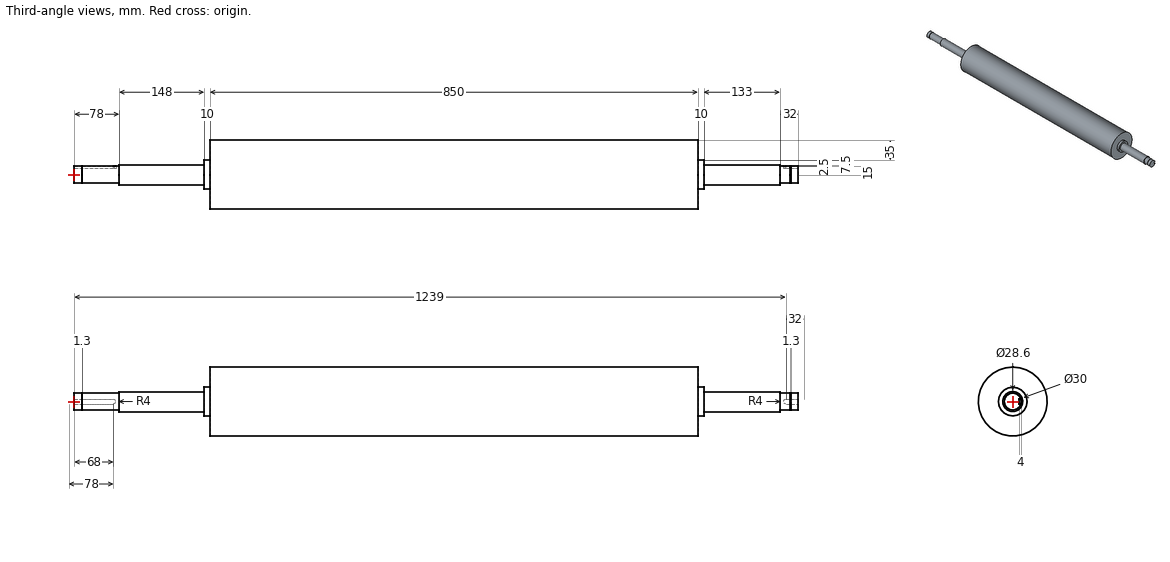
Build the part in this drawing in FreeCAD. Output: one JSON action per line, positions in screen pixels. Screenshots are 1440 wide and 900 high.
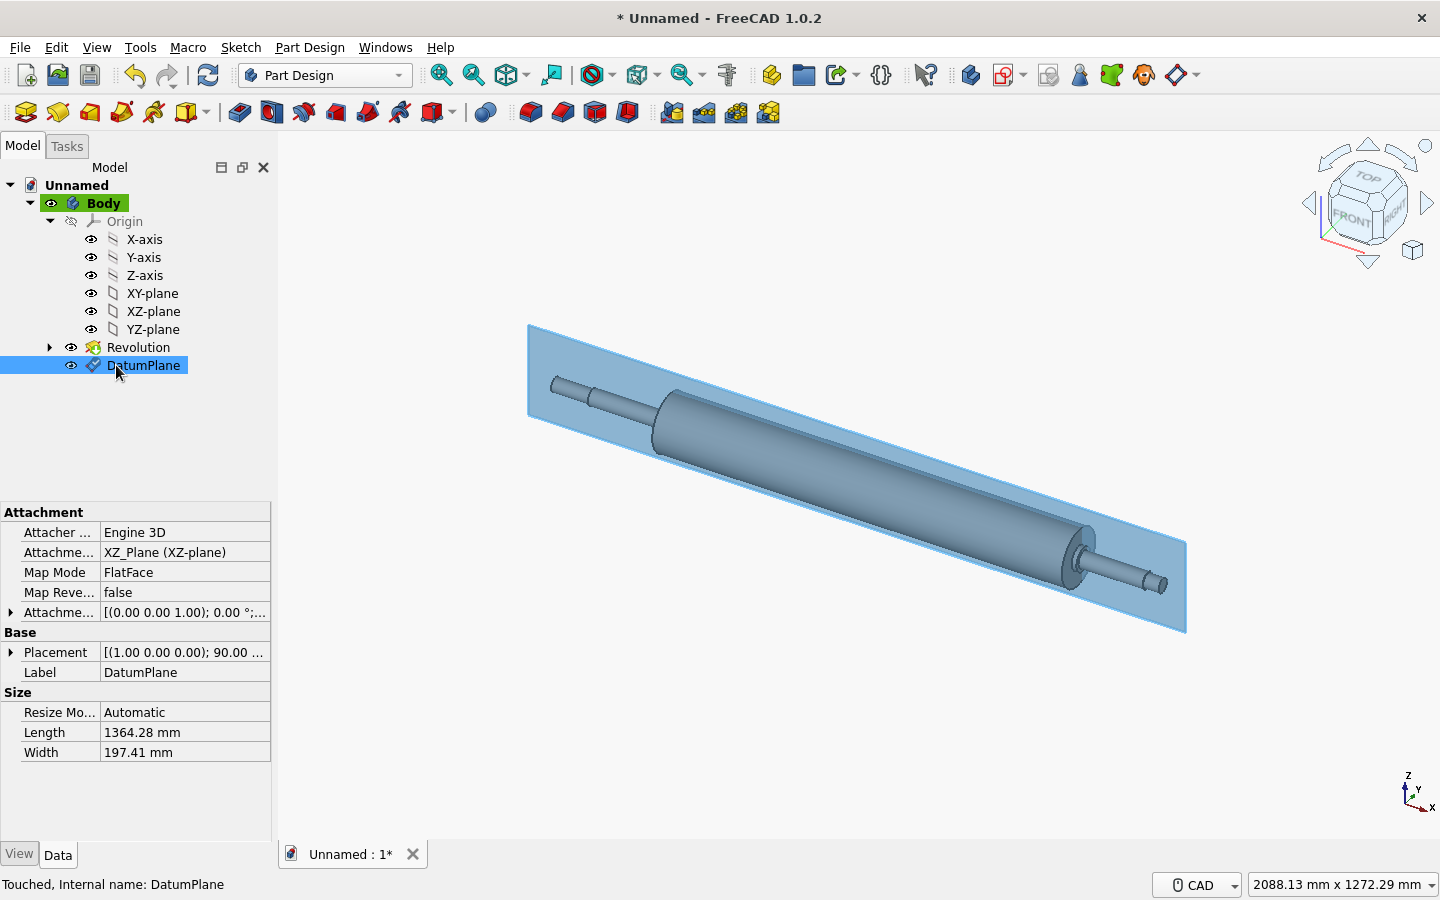
{"action": "left_click", "coordinate": [1004, 76]}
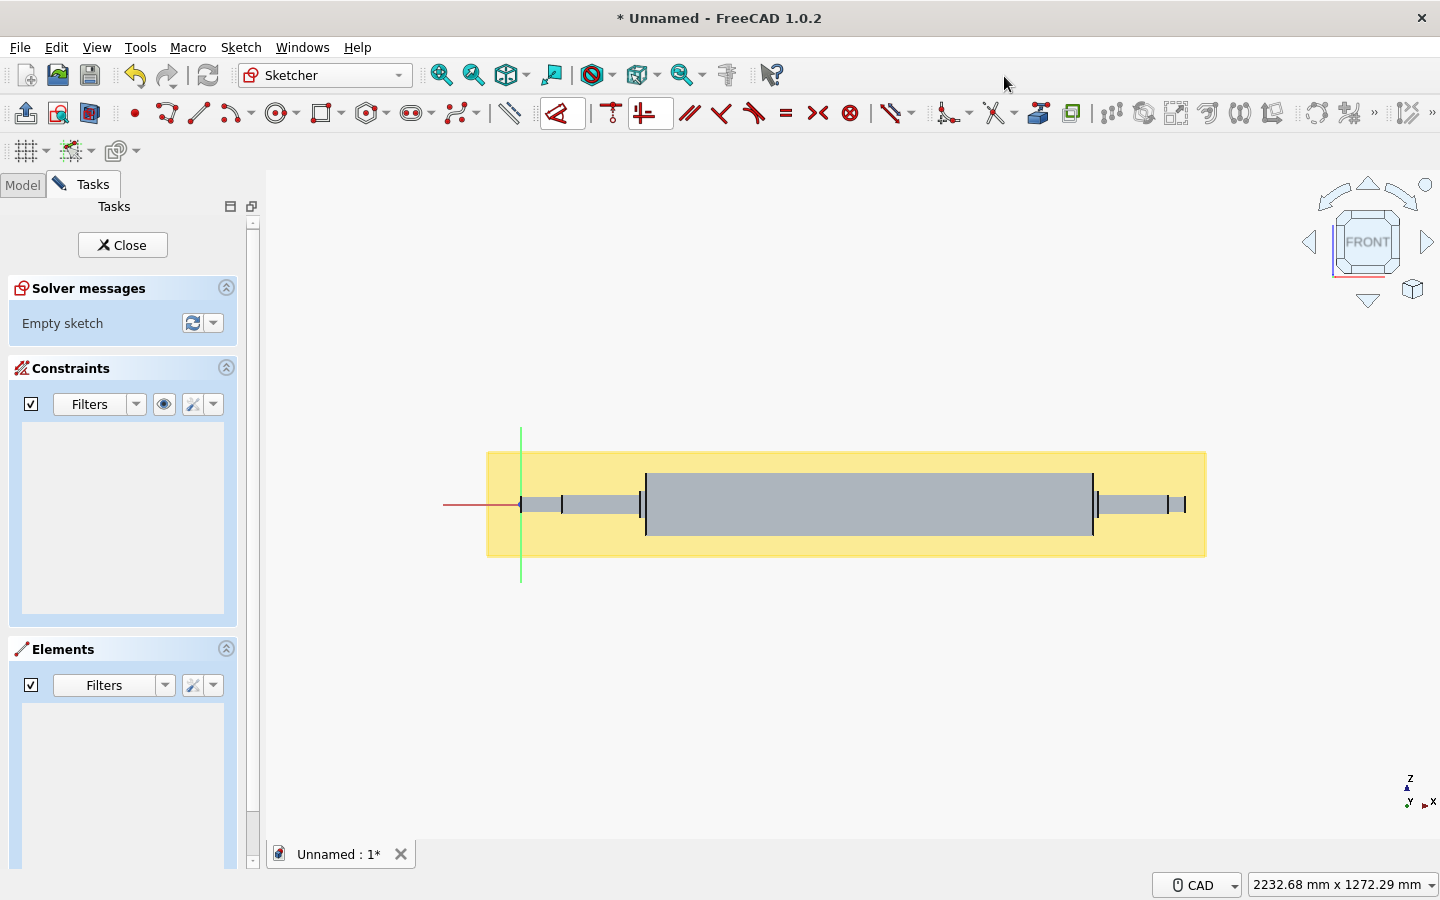
{"action": "left_click", "coordinate": [90, 114]}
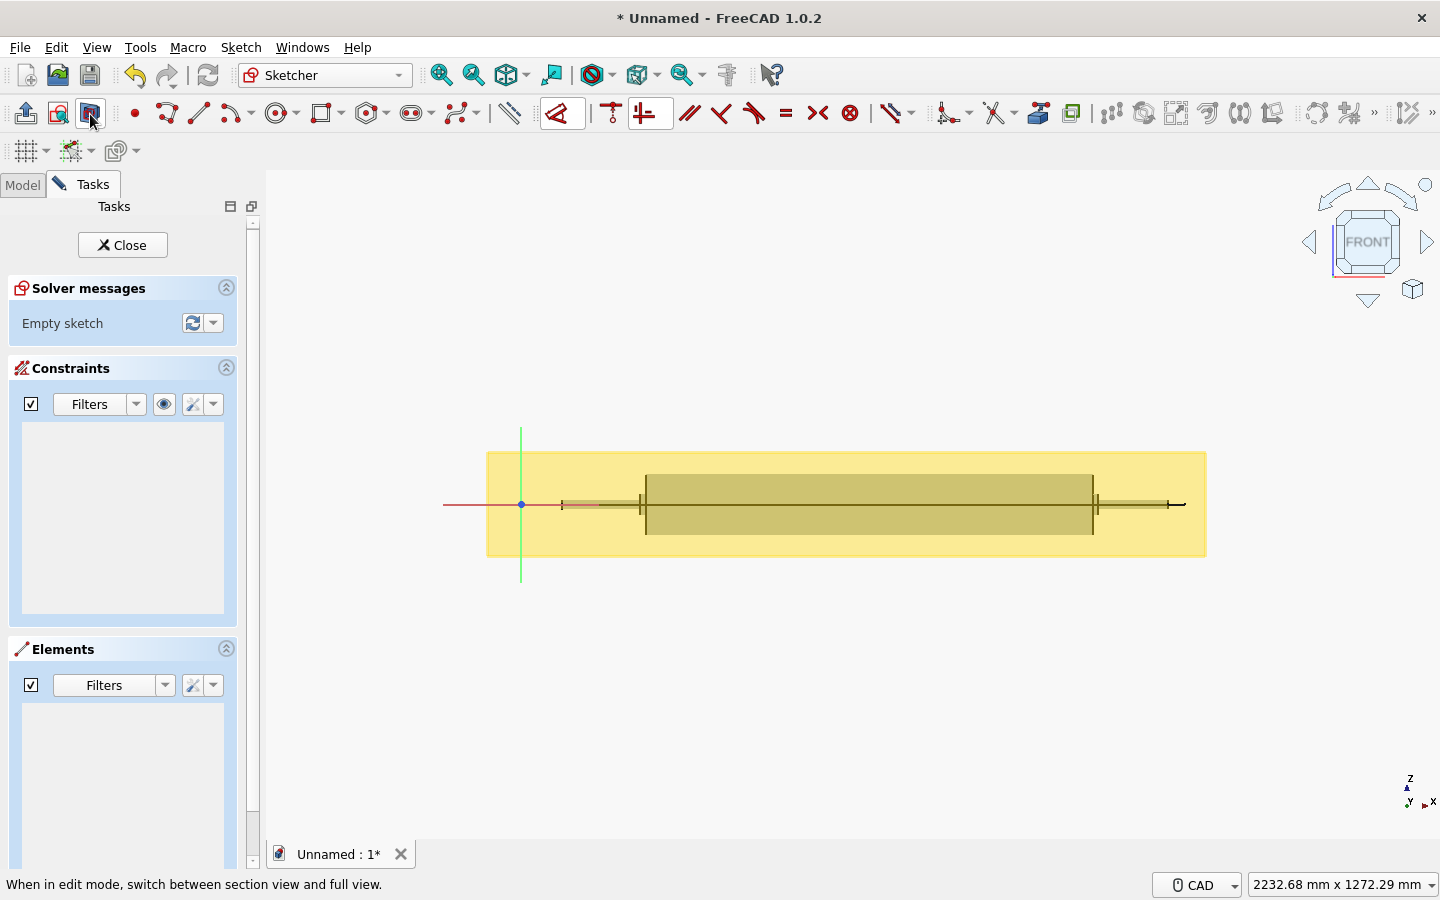
{"action": "scroll", "coordinate": [522, 505], "scroll_direction": "up", "scroll_amount": 14}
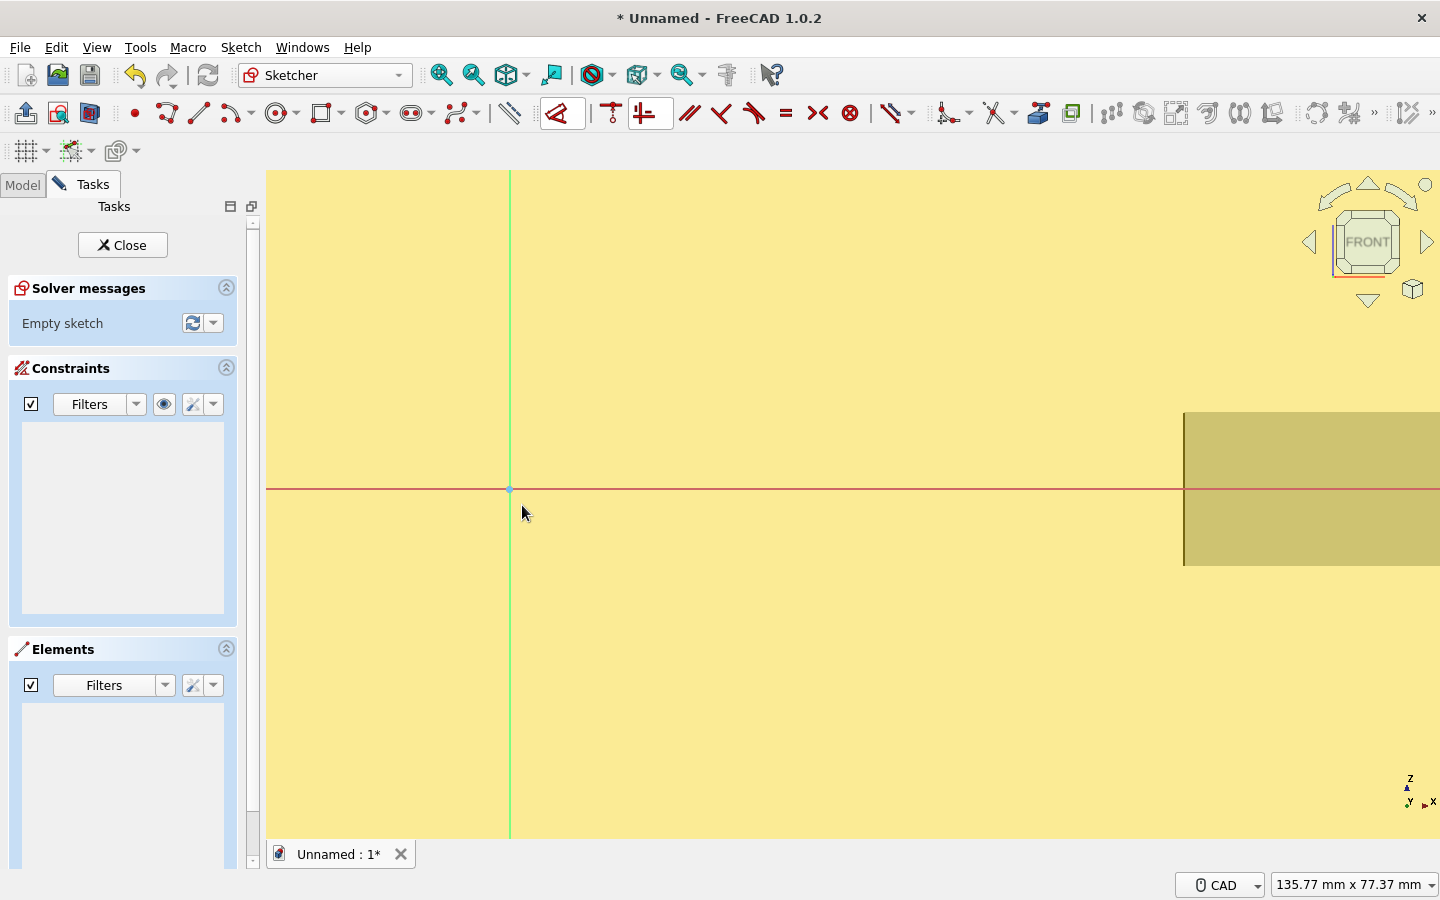
{"action": "key", "text": "g m"}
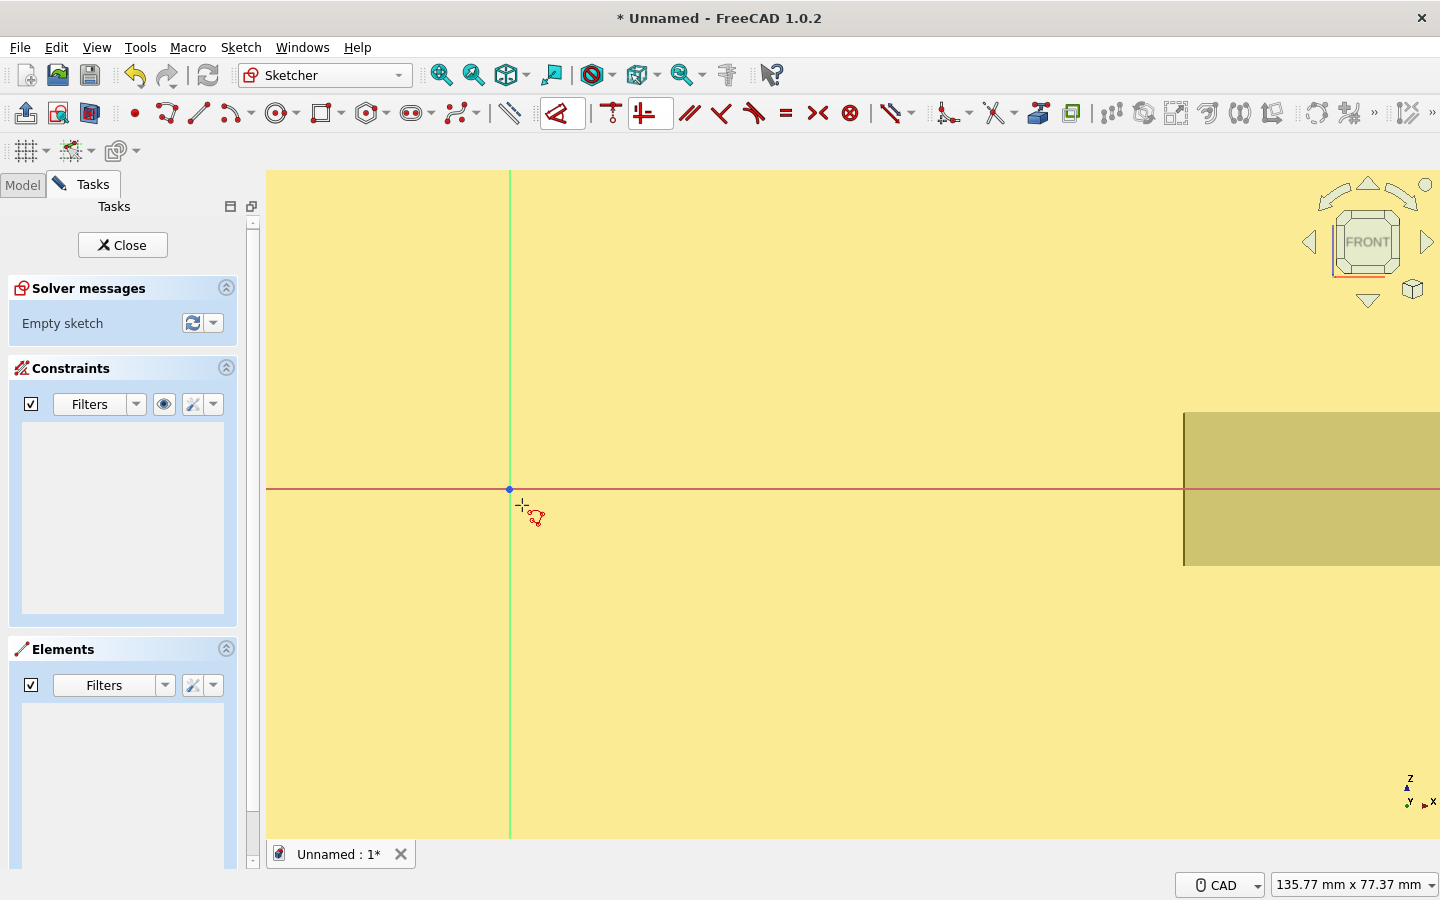
{"action": "left_click", "coordinate": [1098, 524]}
{"action": "left_click", "coordinate": [423, 524]}
{"action": "left_click", "coordinate": [423, 454]}
{"action": "left_click", "coordinate": [1098, 454]}
{"action": "right_click", "coordinate": [1098, 454]}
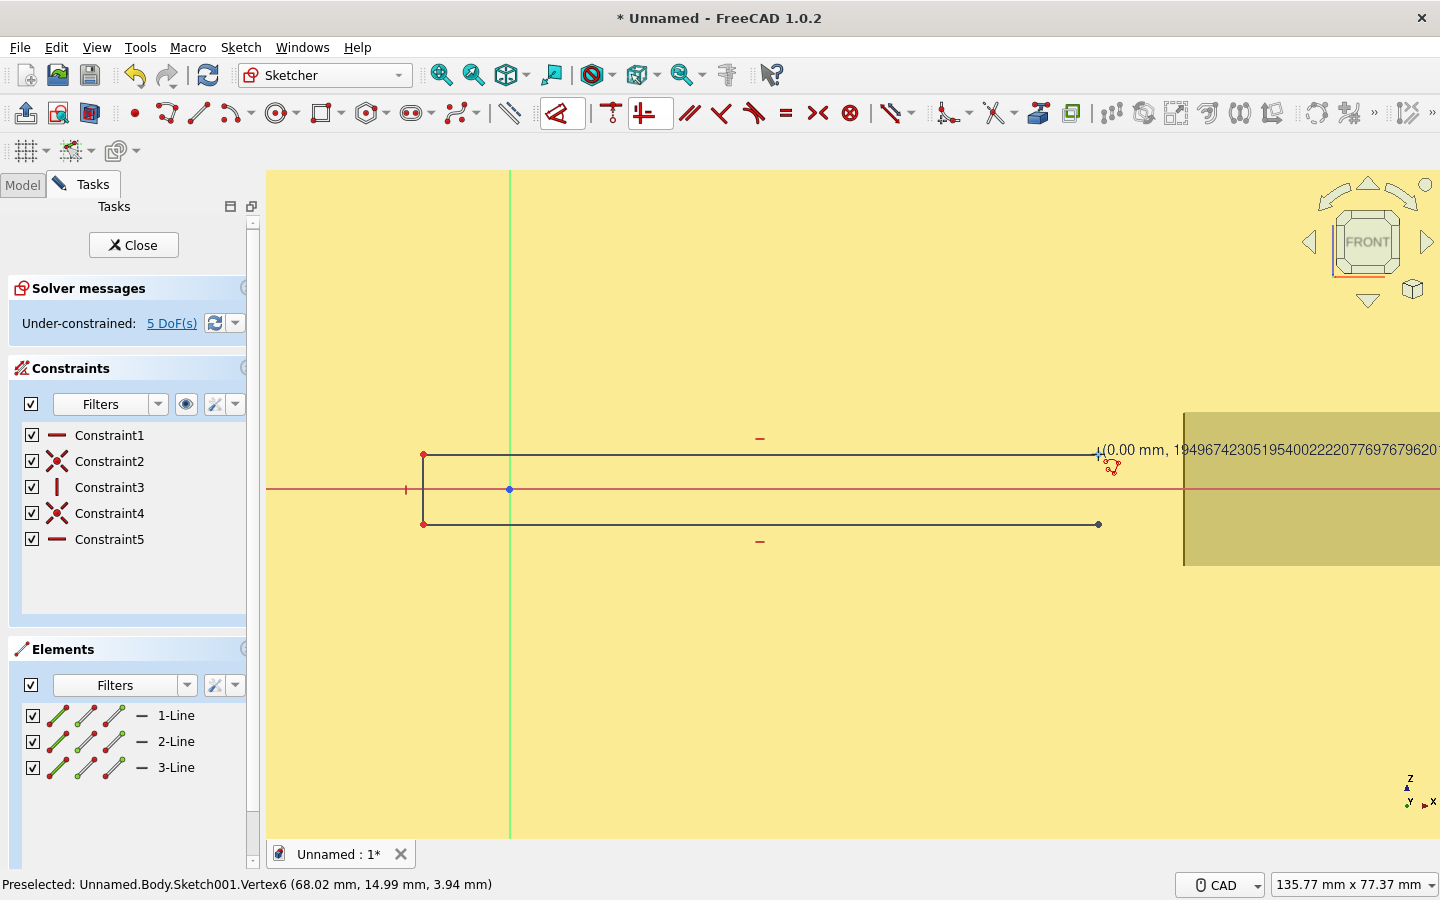
{"action": "left_click", "coordinate": [254, 114]}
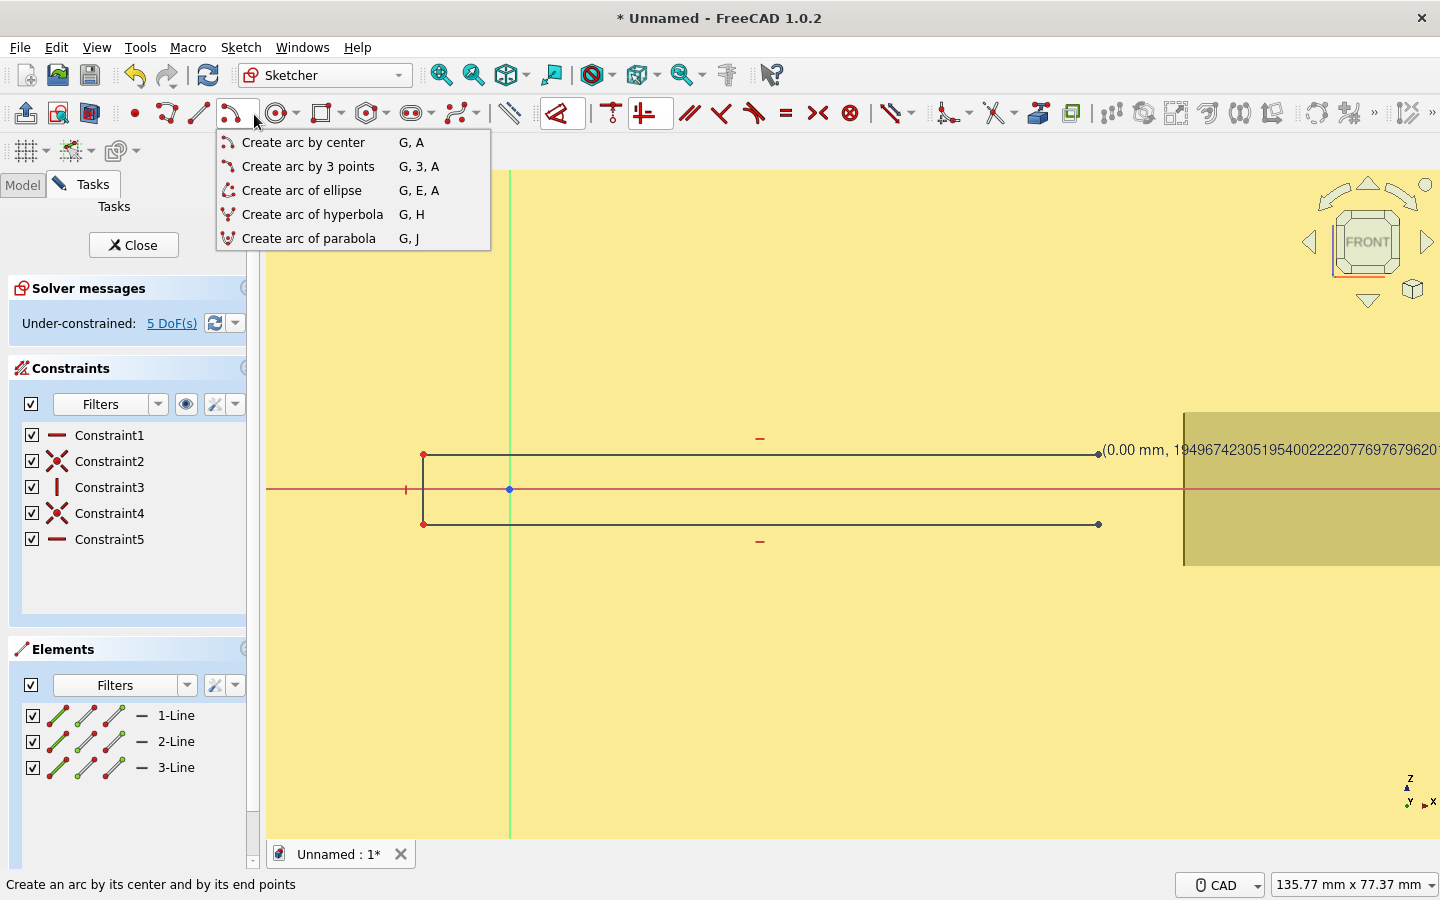
{"action": "left_click", "coordinate": [354, 166]}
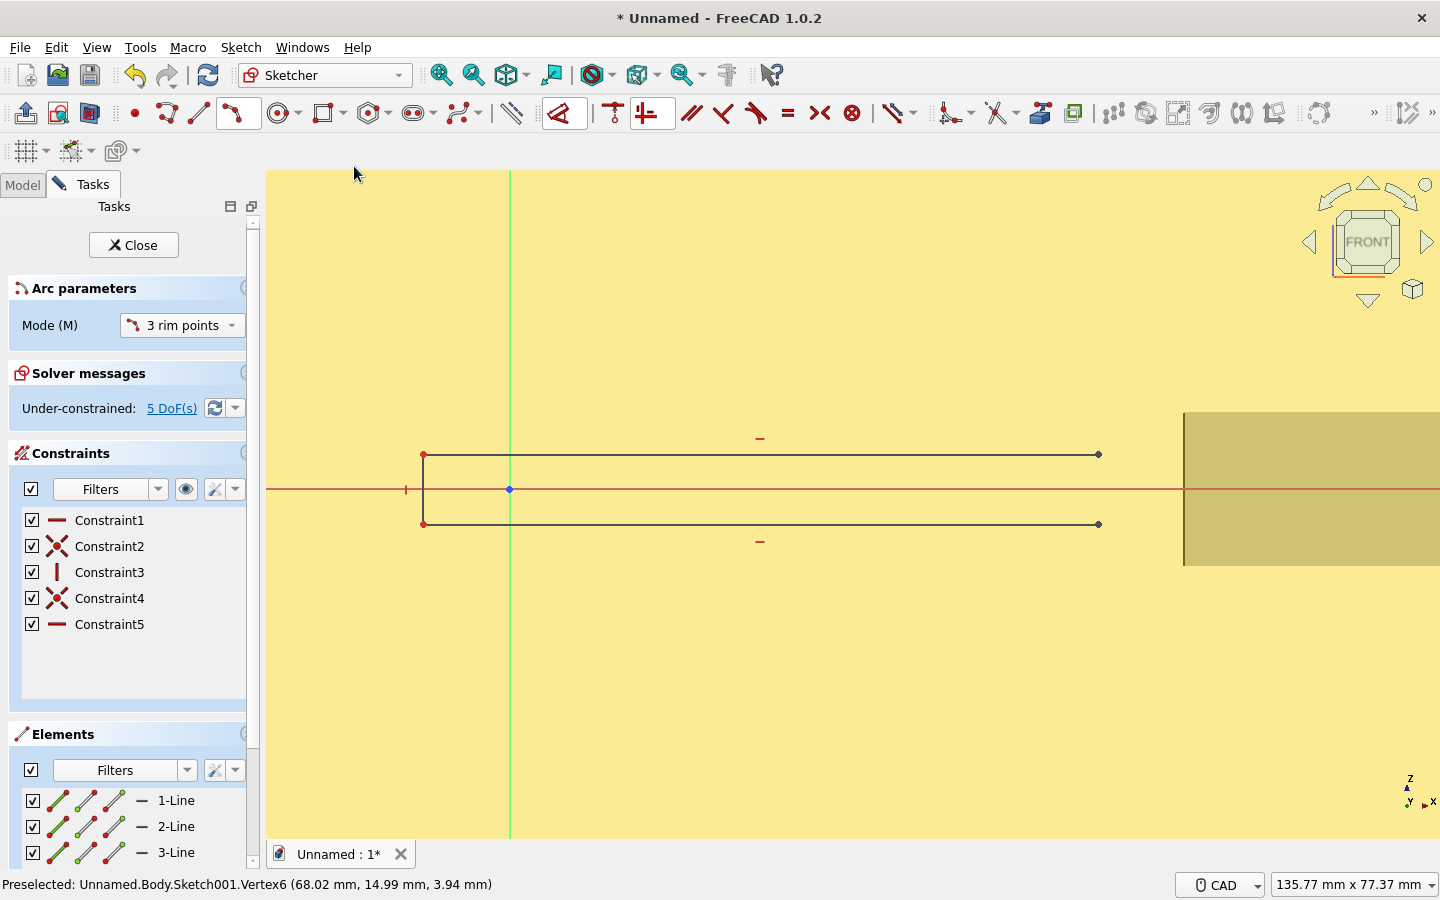
{"action": "left_click", "coordinate": [1098, 455]}
{"action": "left_click", "coordinate": [1098, 525]}
{"action": "left_click", "coordinate": [1126, 509]}
{"action": "key", "text": "Escape"}